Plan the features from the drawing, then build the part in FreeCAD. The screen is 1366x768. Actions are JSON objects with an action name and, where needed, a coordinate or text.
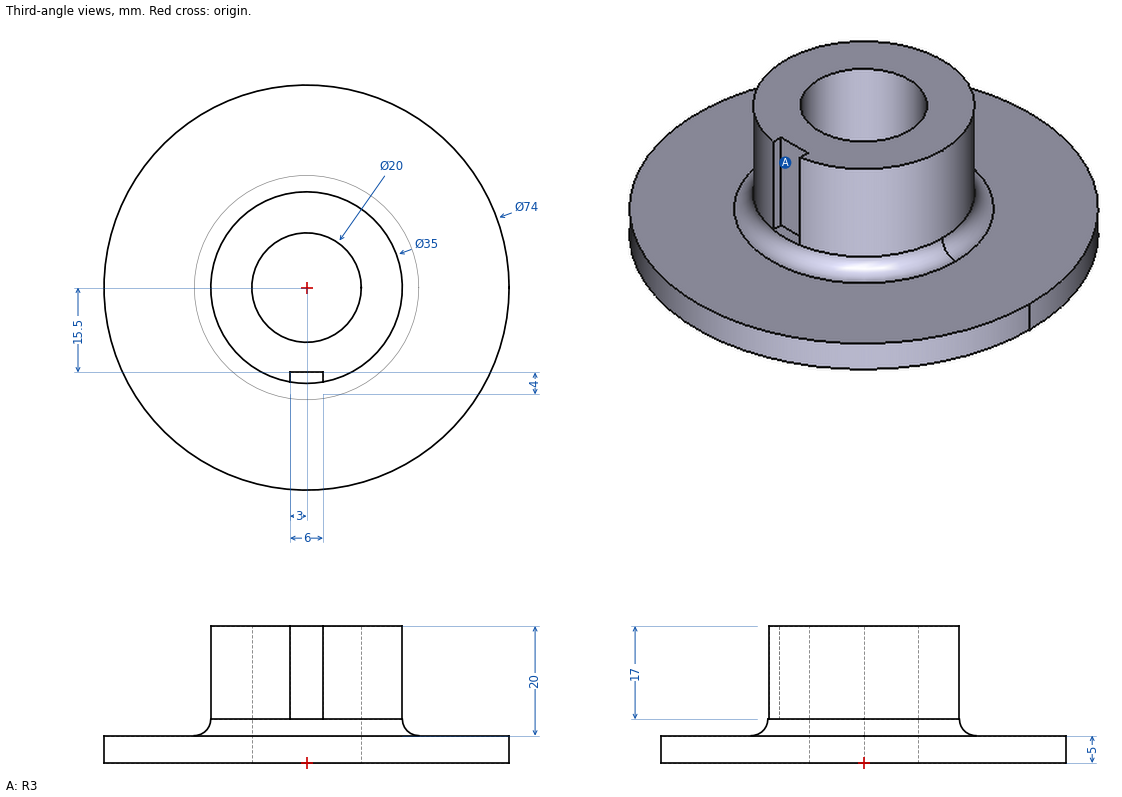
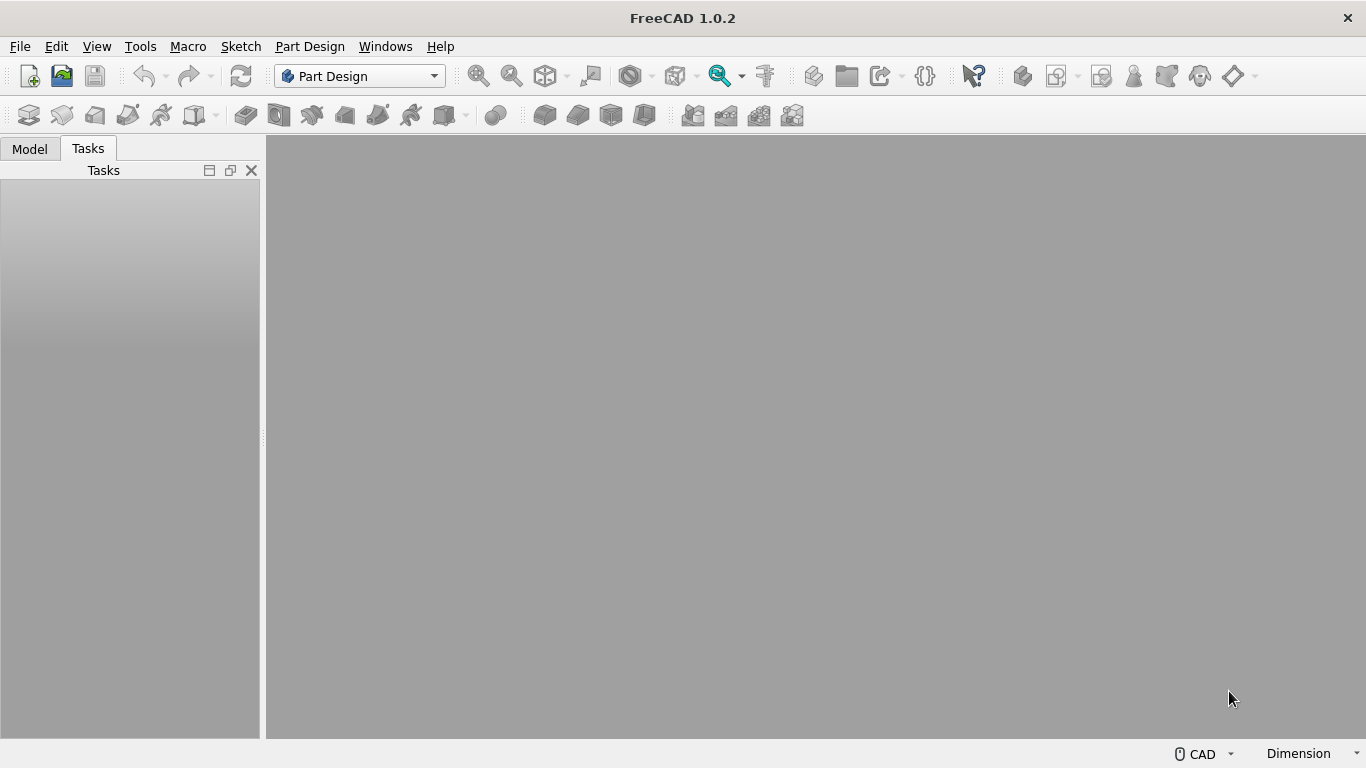
{"action": "left_click", "coordinate": [29, 76]}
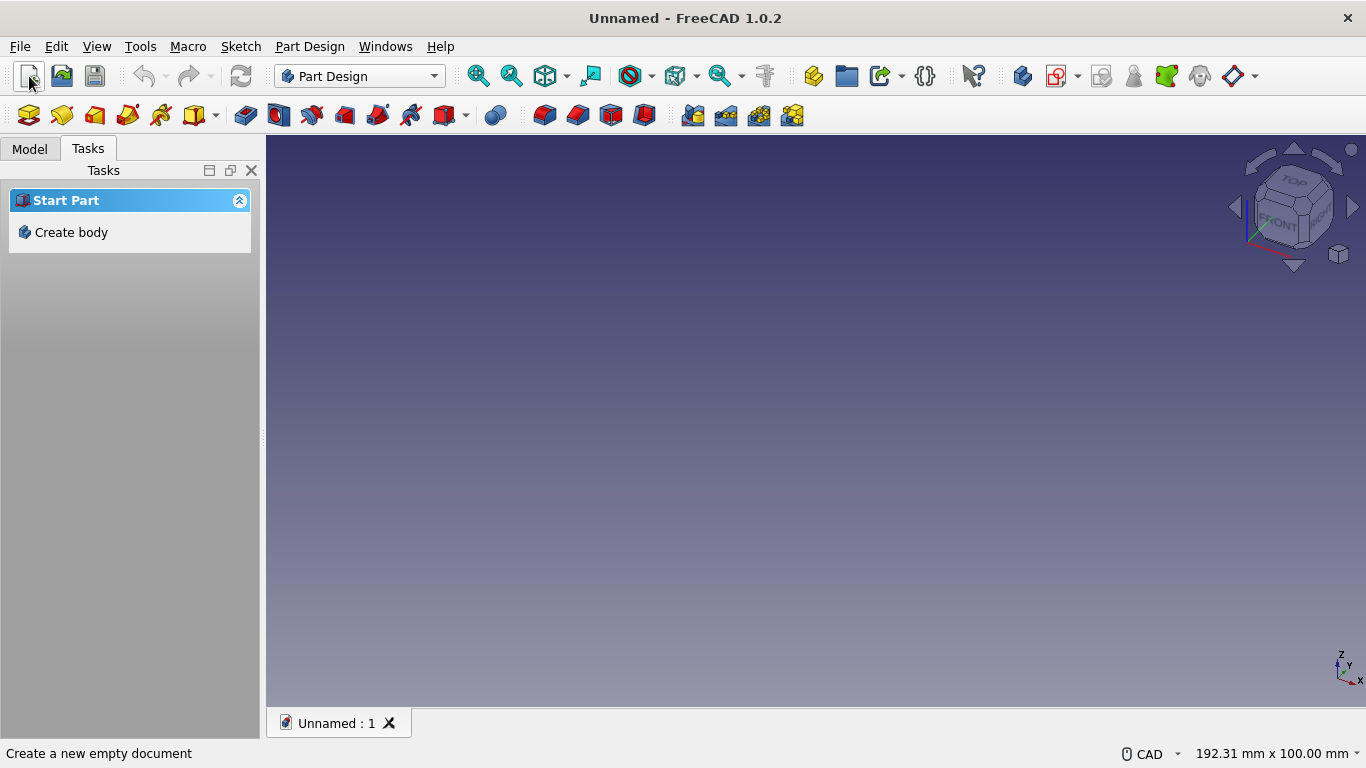
{"action": "left_click", "coordinate": [1056, 76]}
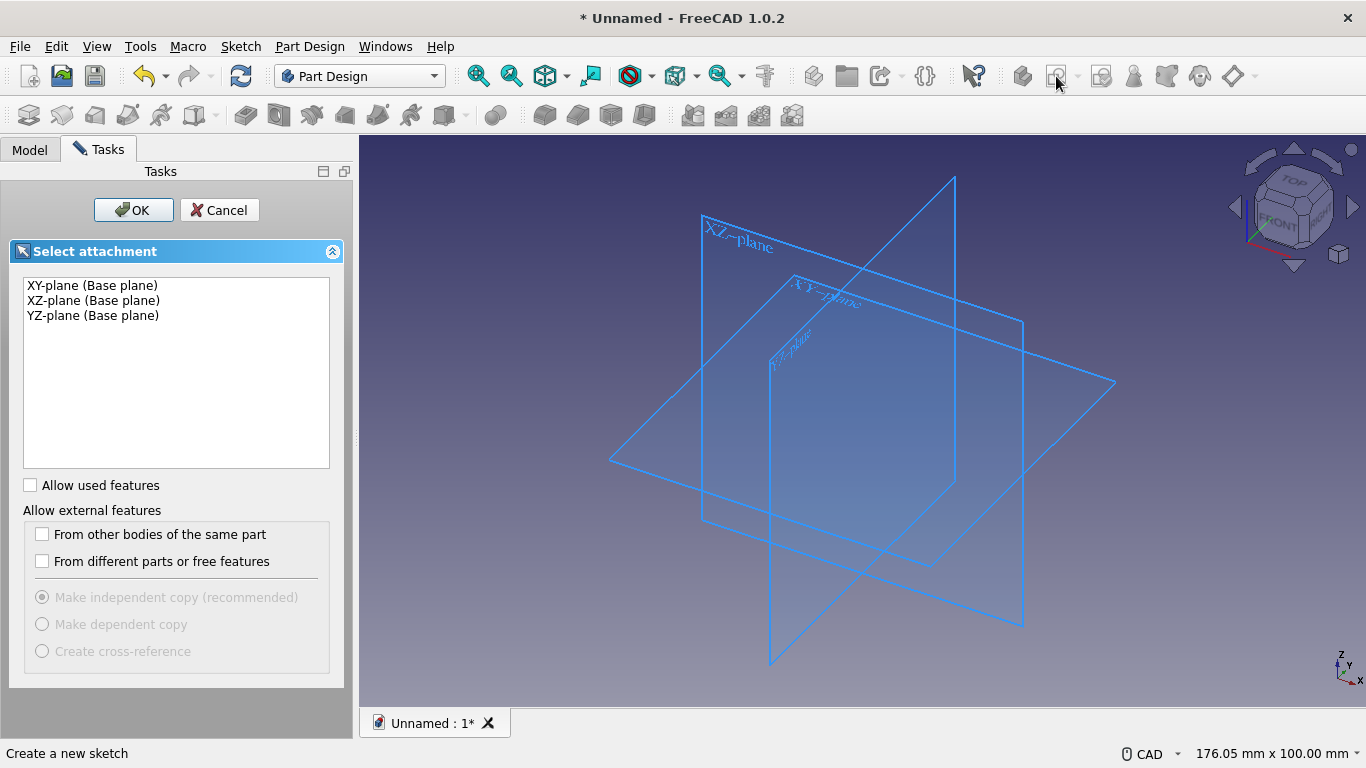
{"action": "left_click", "coordinate": [84, 286]}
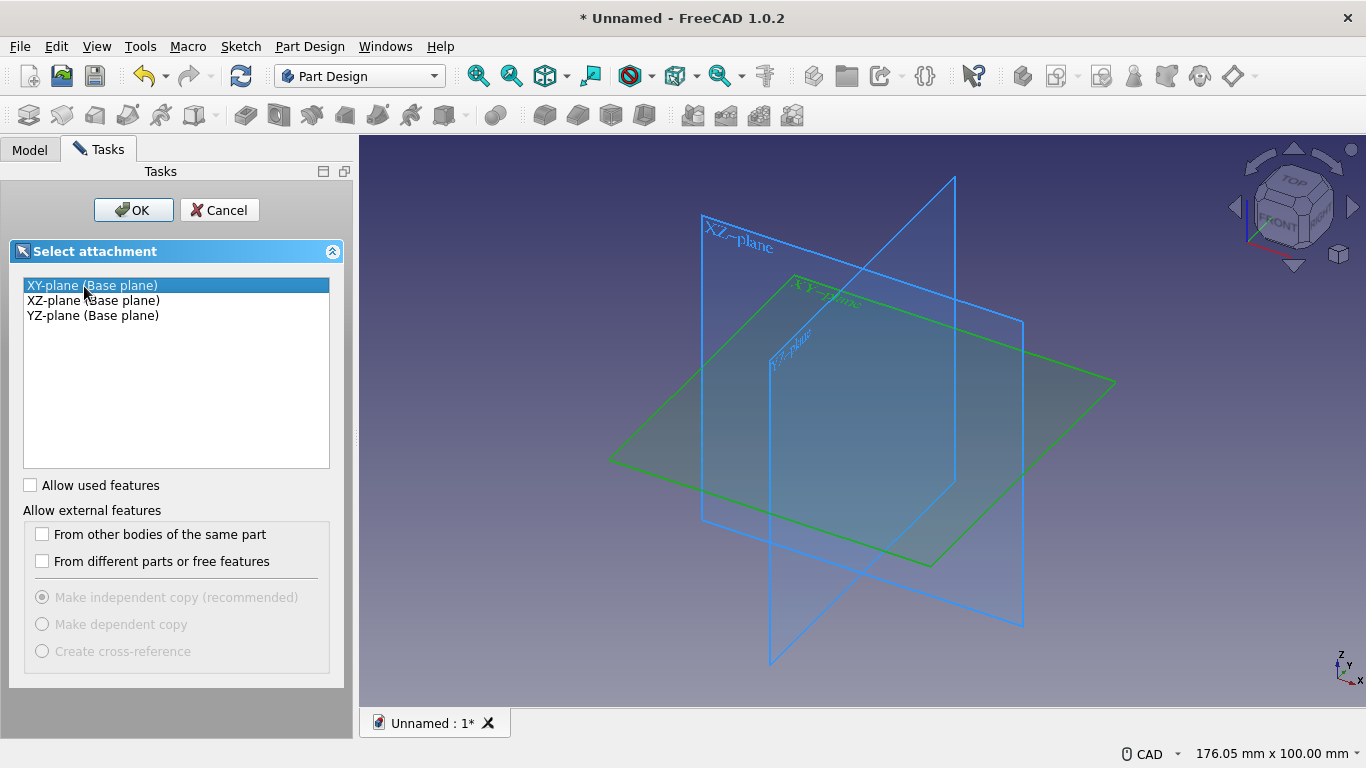
{"action": "left_click", "coordinate": [134, 210]}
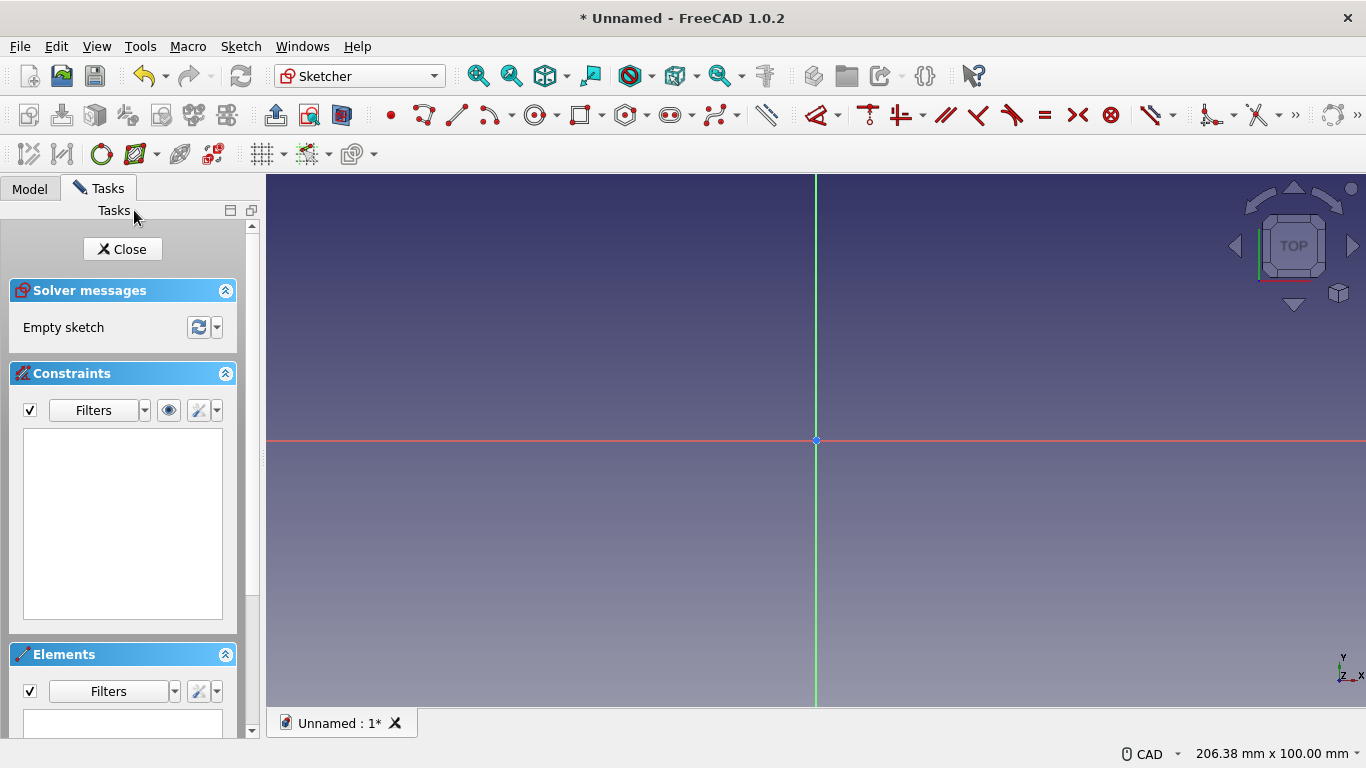
{"action": "left_click", "coordinate": [534, 116]}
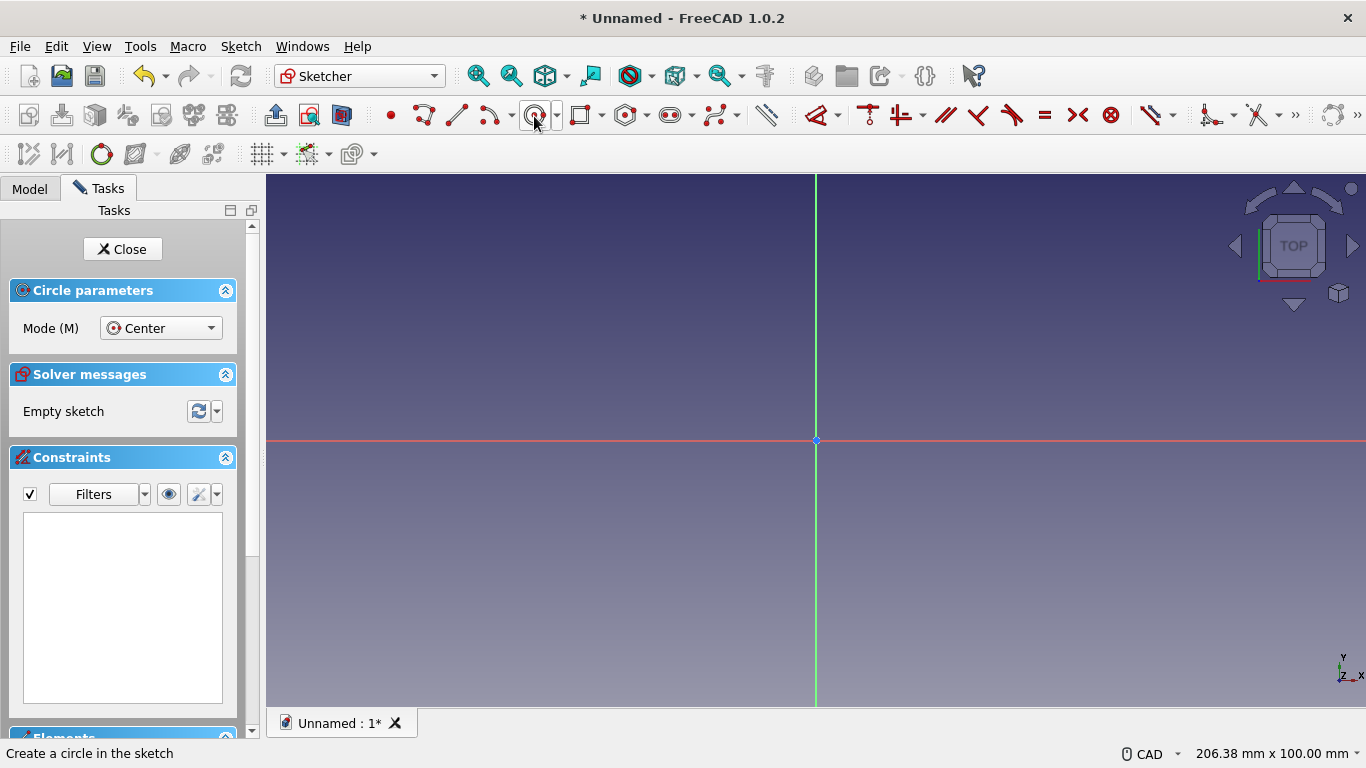
{"action": "left_click", "coordinate": [816, 440]}
{"action": "mouse_move", "coordinate": [955, 301]}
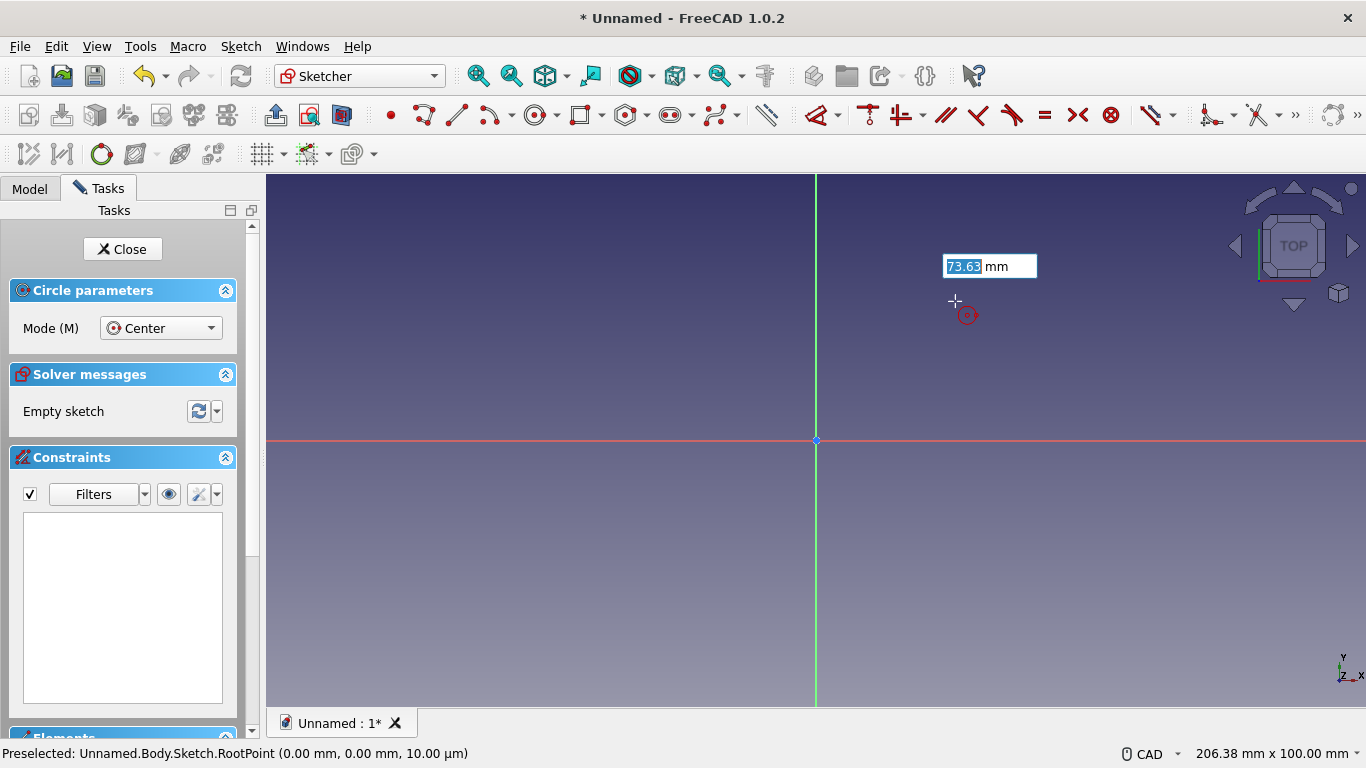
{"action": "type", "text": "74"}
{"action": "key", "text": "Return"}
{"action": "key", "text": "Escape"}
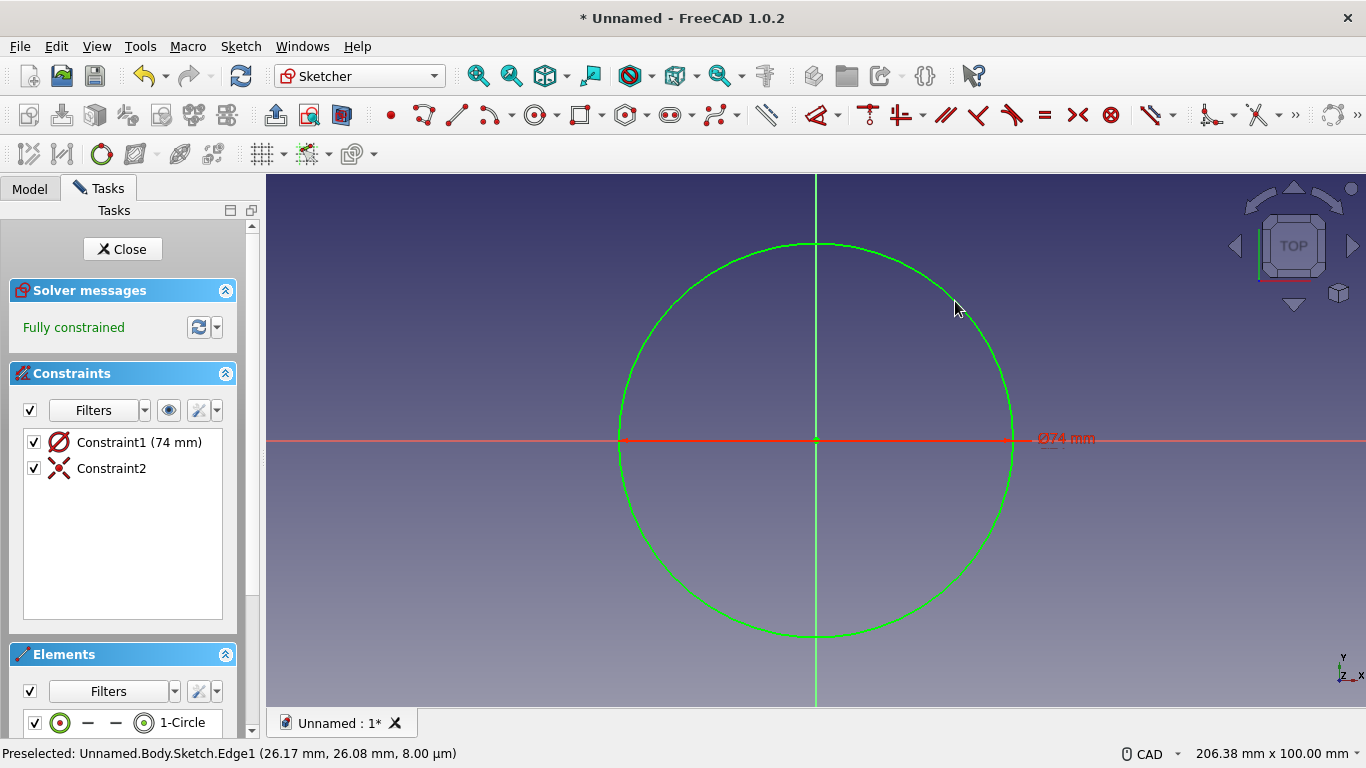
{"action": "left_click", "coordinate": [123, 249]}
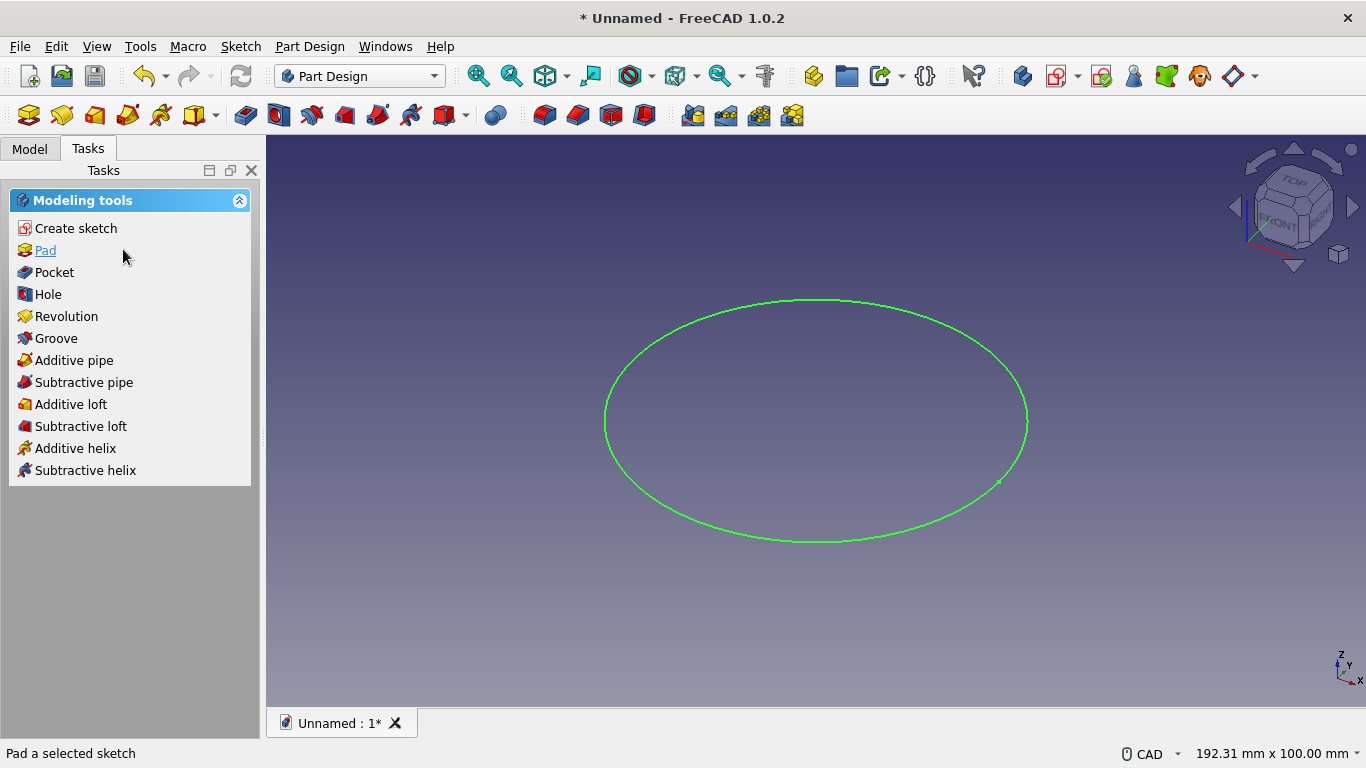
{"action": "left_click", "coordinate": [29, 116]}